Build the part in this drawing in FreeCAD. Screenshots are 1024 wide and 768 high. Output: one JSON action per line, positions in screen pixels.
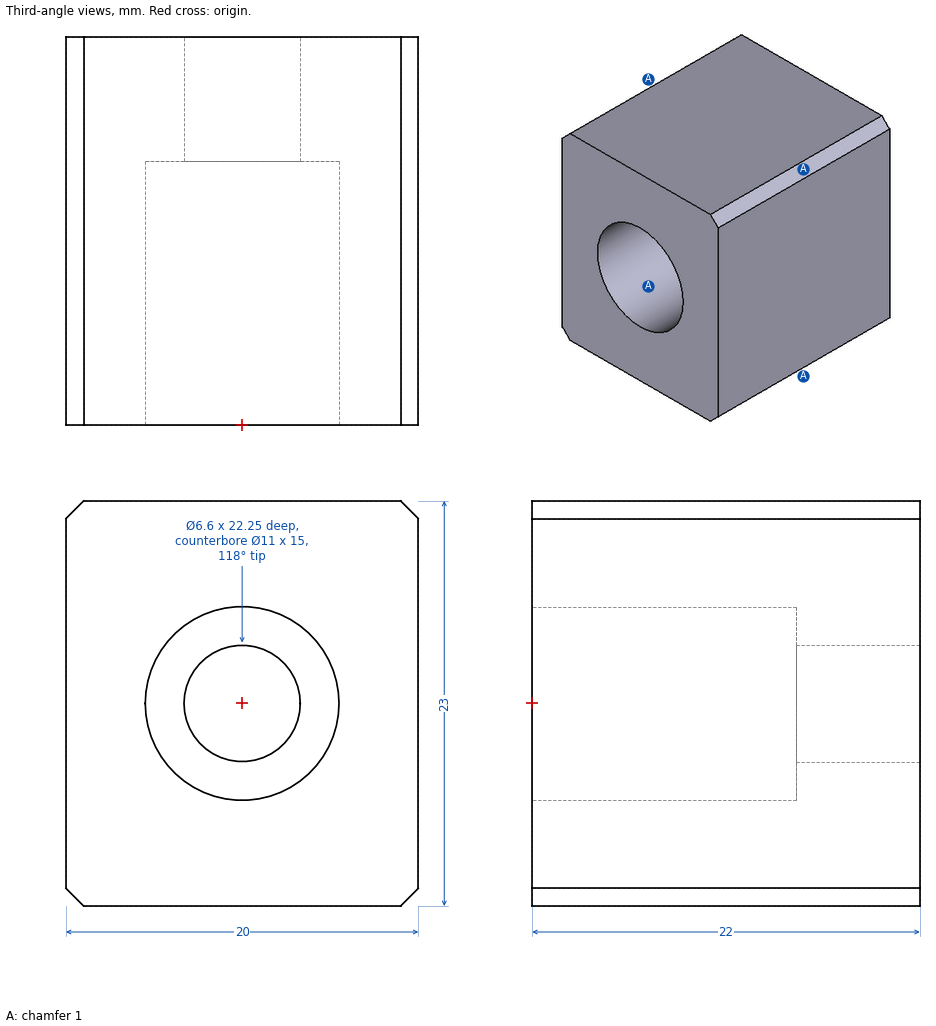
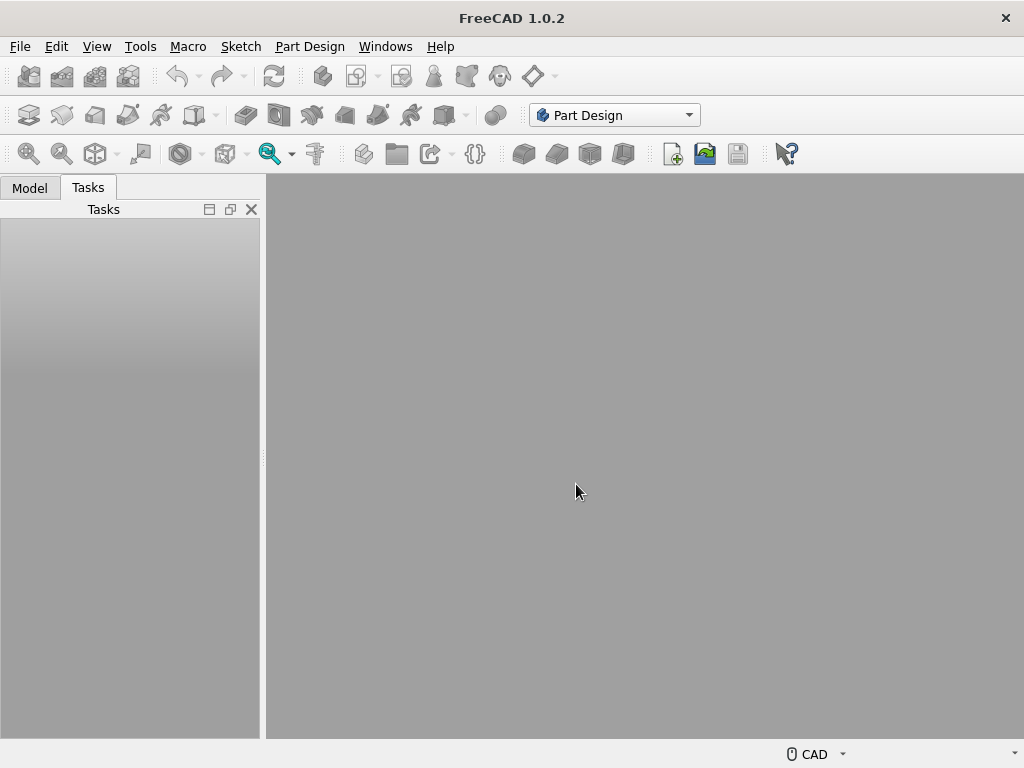
{"action": "key", "text": "ctrl+n"}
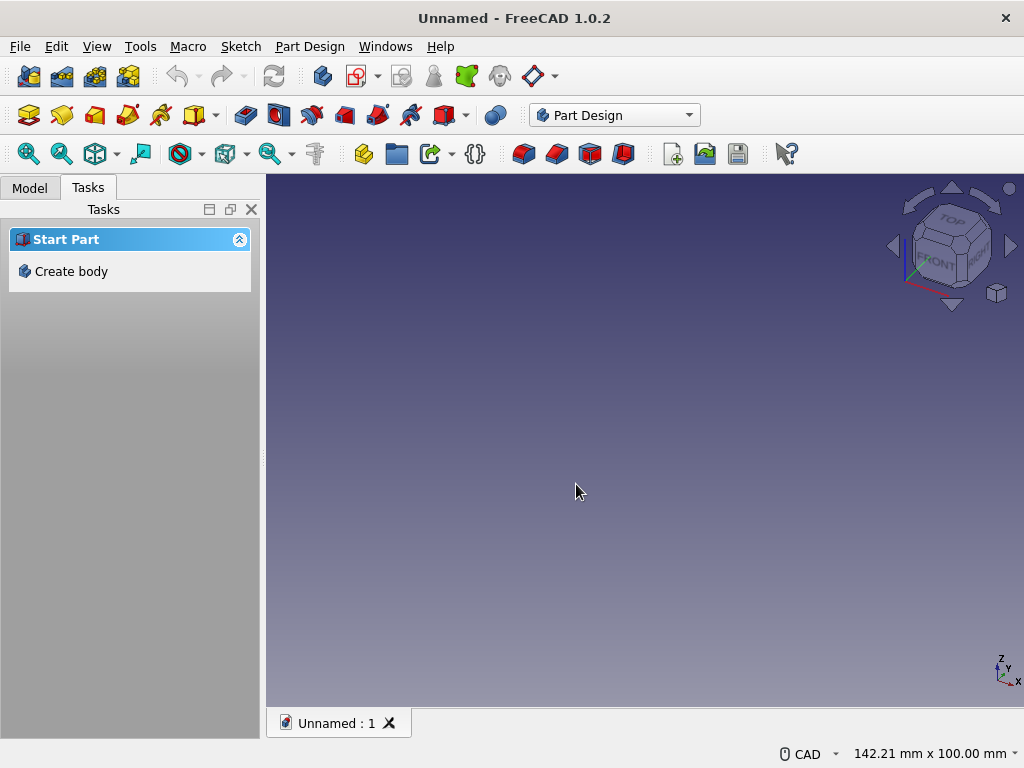
{"action": "left_click", "coordinate": [356, 76]}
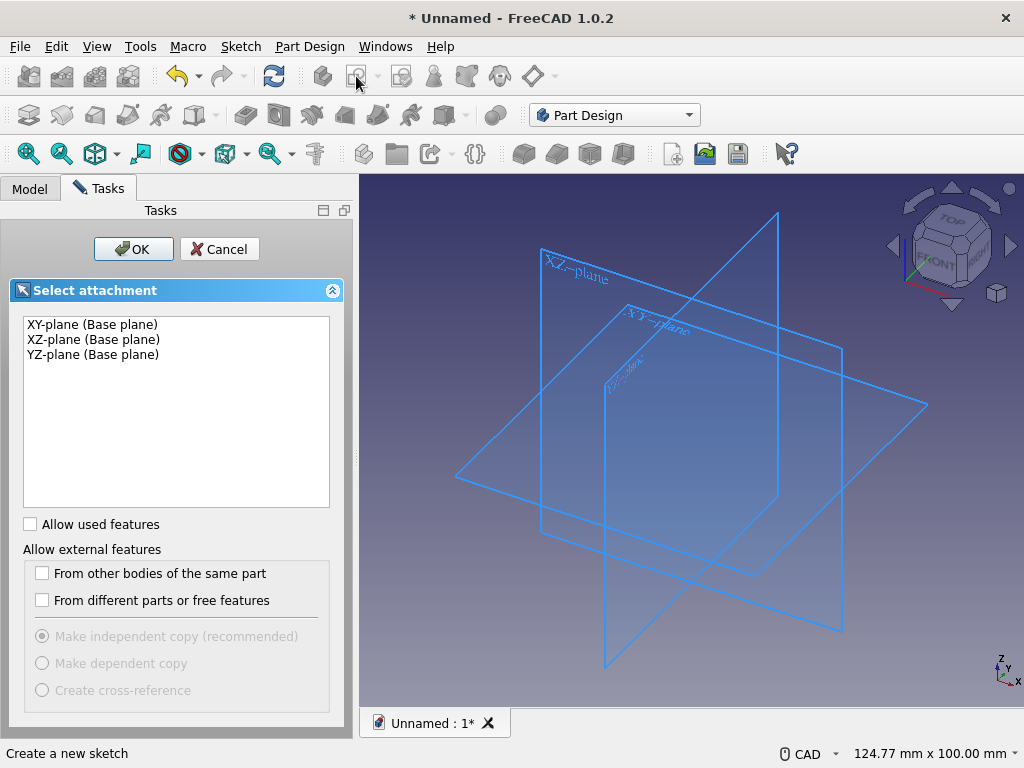
{"action": "left_click", "coordinate": [84, 340]}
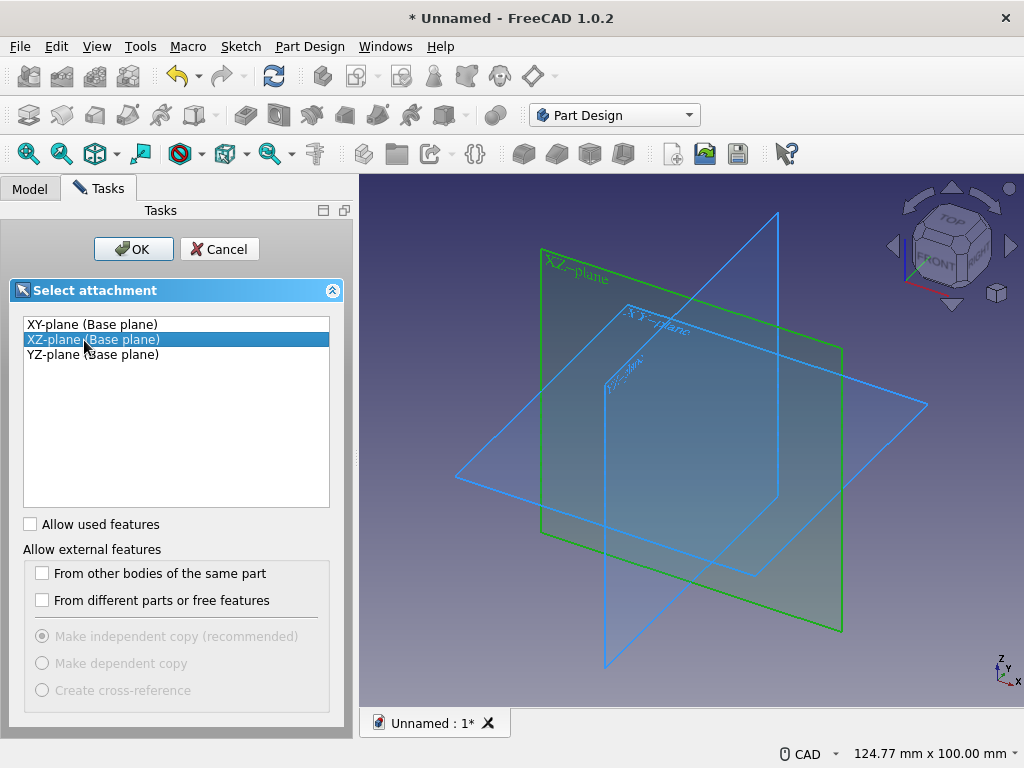
{"action": "left_click", "coordinate": [134, 249]}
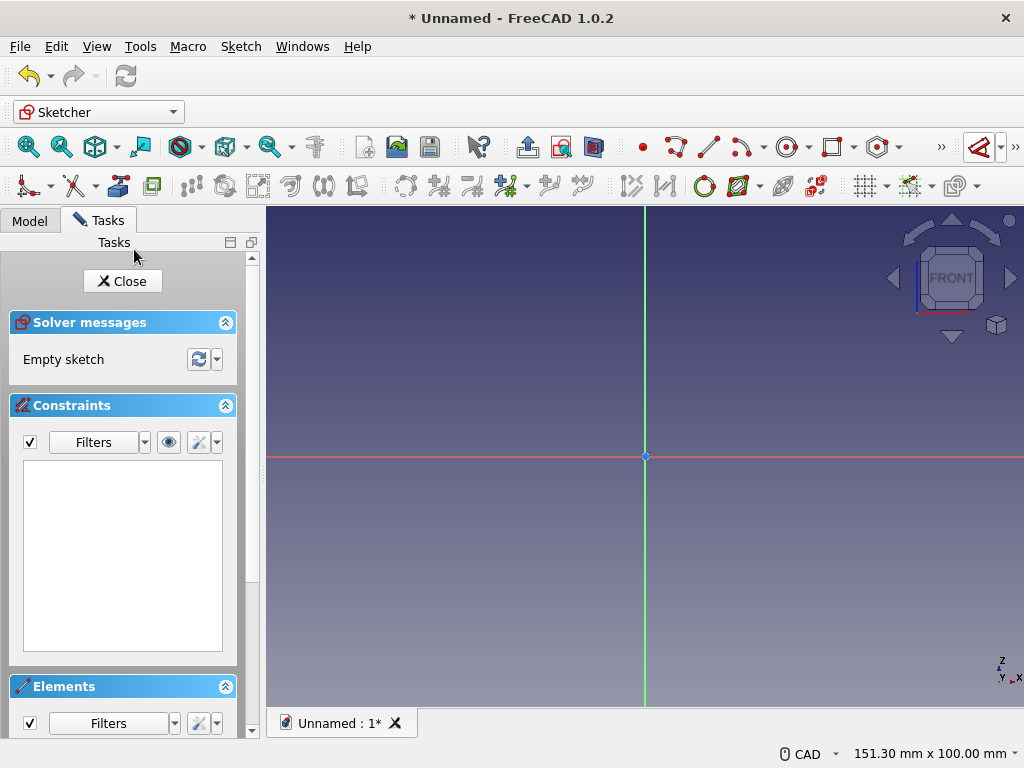
{"action": "scroll", "coordinate": [685, 456], "scroll_direction": "up", "scroll_amount": 5}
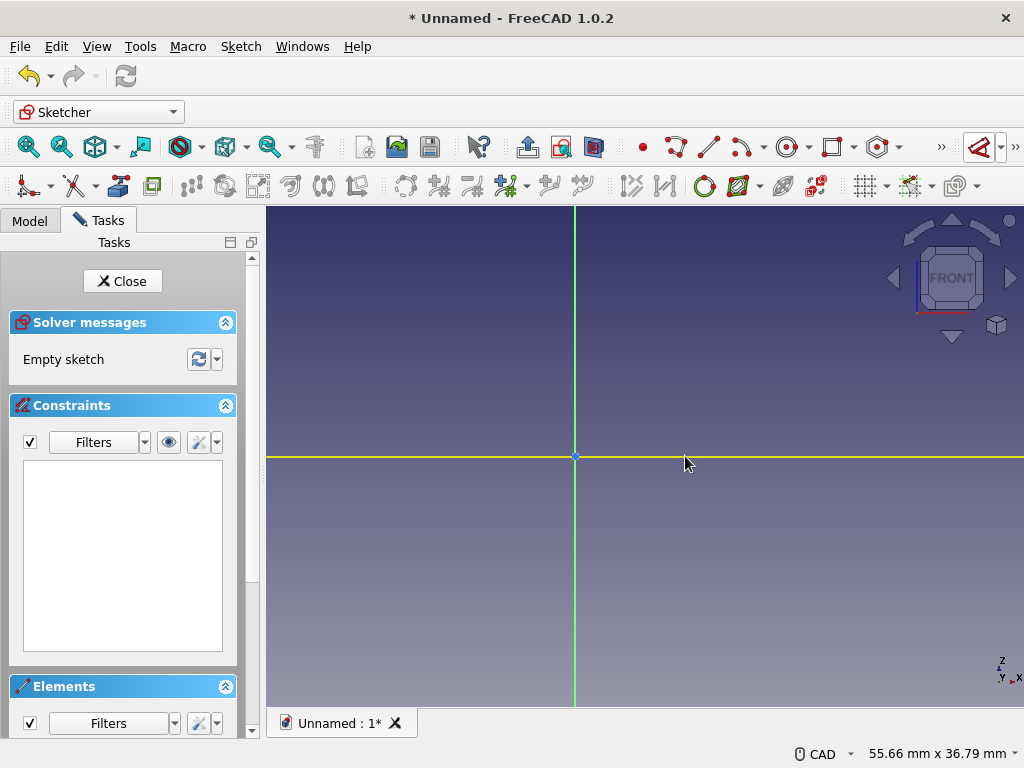
{"action": "key", "text": "g v"}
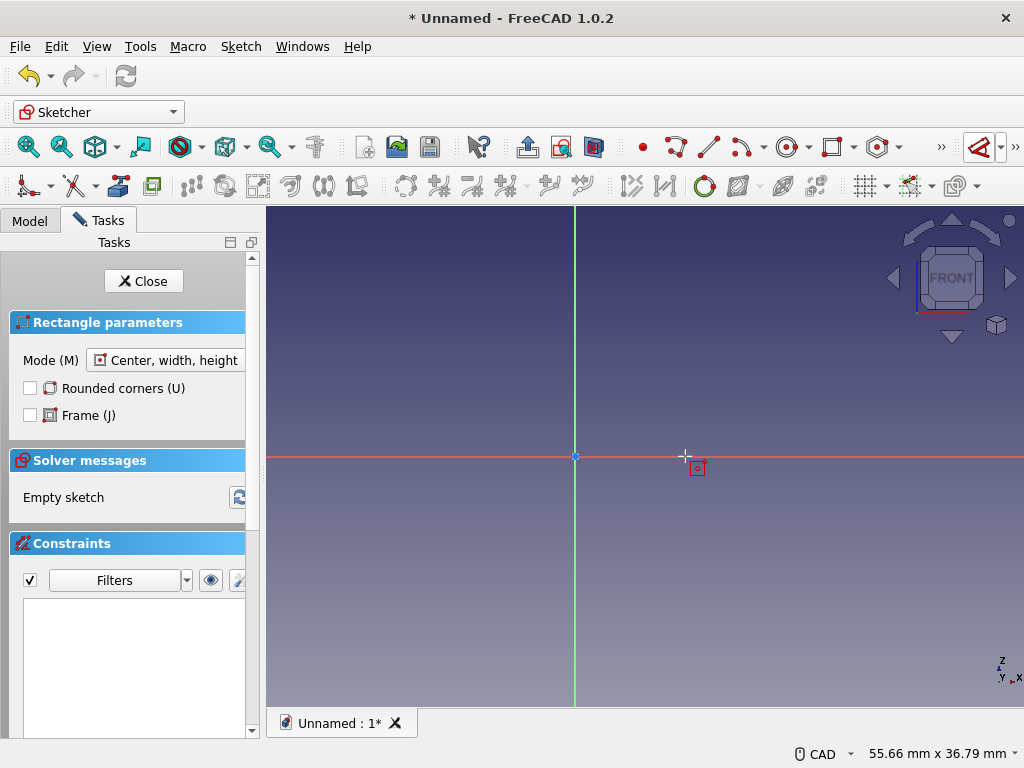
{"action": "left_click", "coordinate": [575, 456]}
{"action": "mouse_move", "coordinate": [712, 300]}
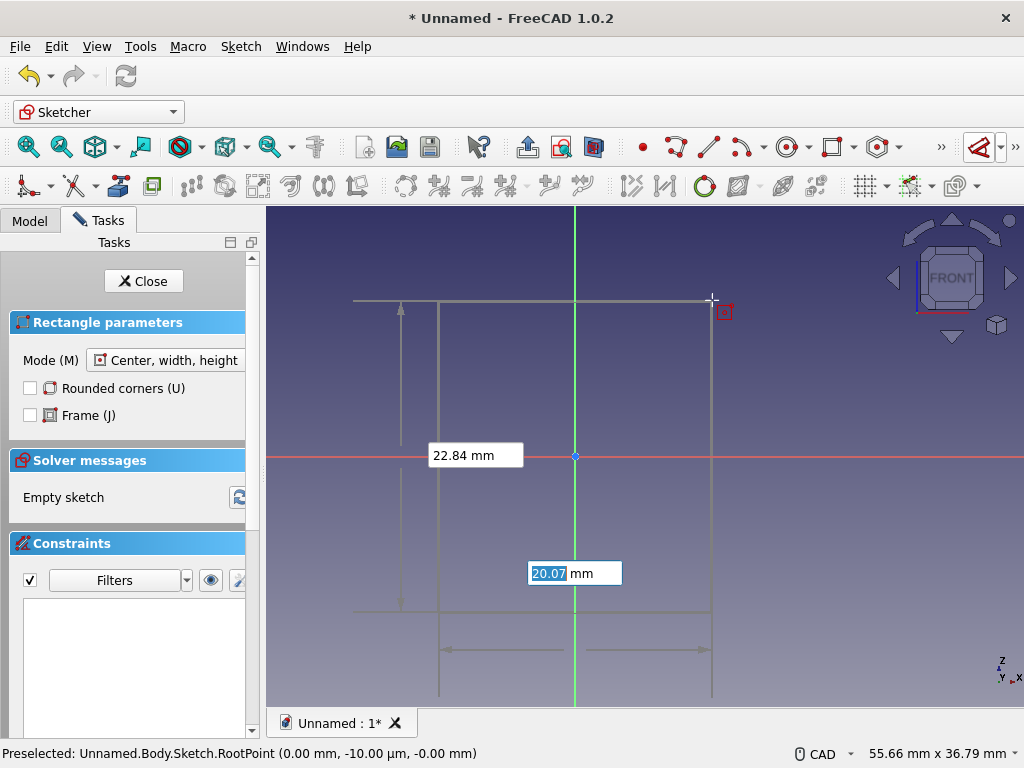
{"action": "type", "text": "20"}
{"action": "key", "text": "Tab"}
{"action": "type", "text": "23"}
{"action": "key", "text": "Return"}
{"action": "key", "text": "Escape"}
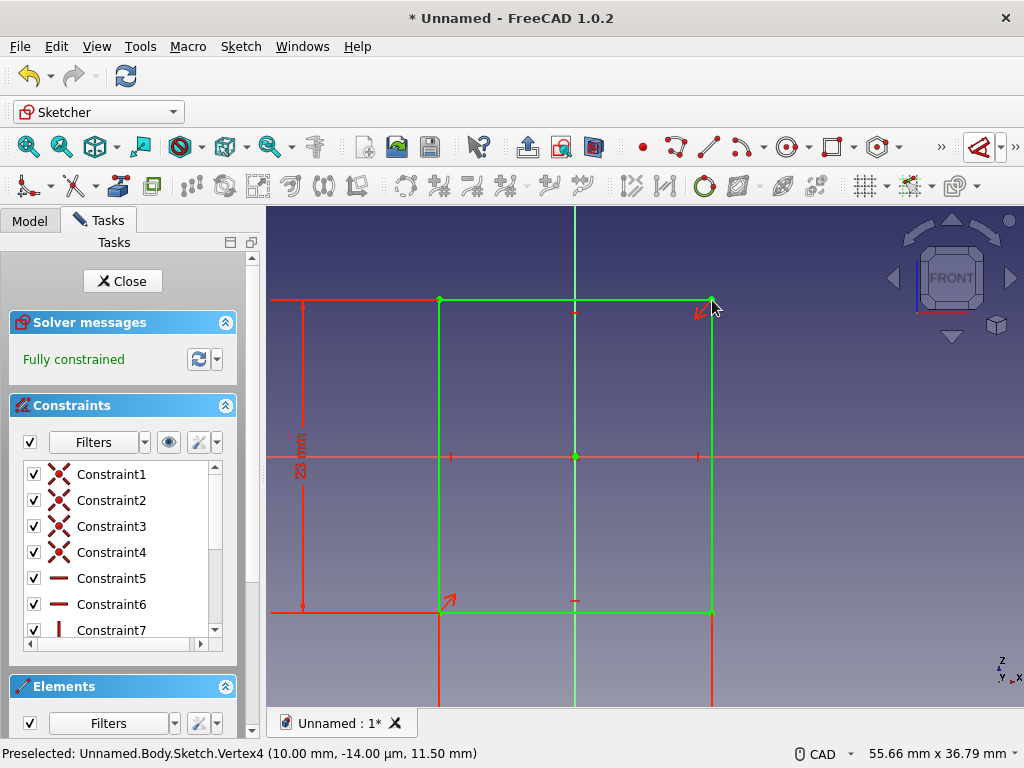
{"action": "left_click", "coordinate": [123, 281]}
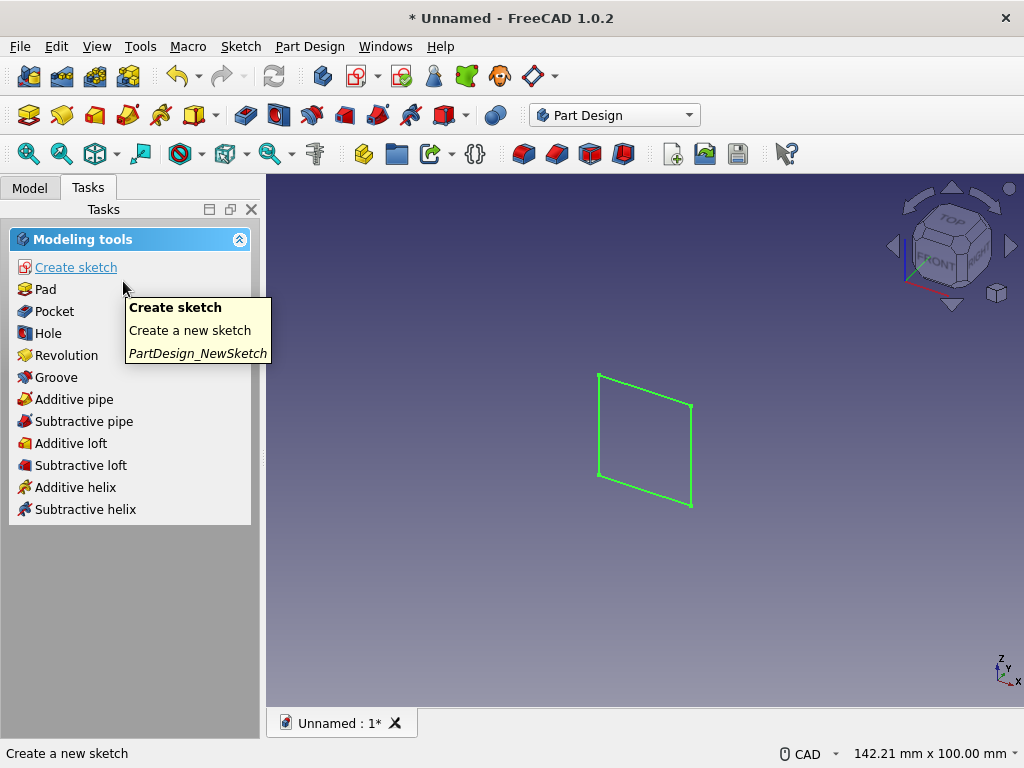
{"action": "left_click", "coordinate": [29, 116]}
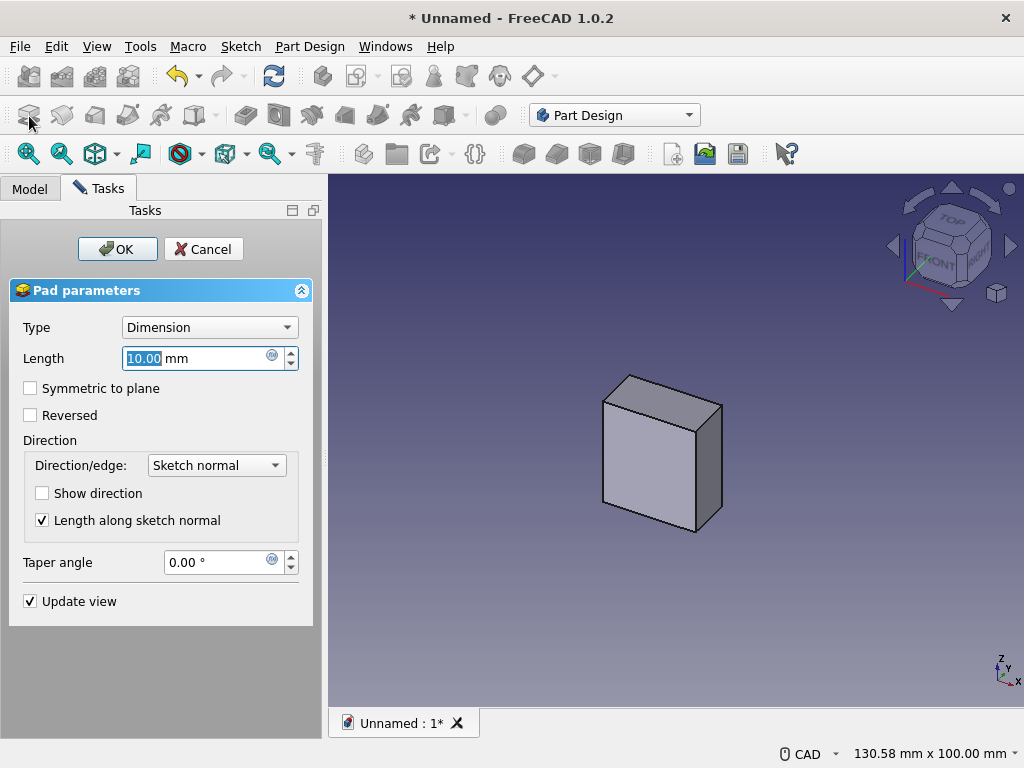
{"action": "type", "text": "22"}
{"action": "key", "text": "Tab"}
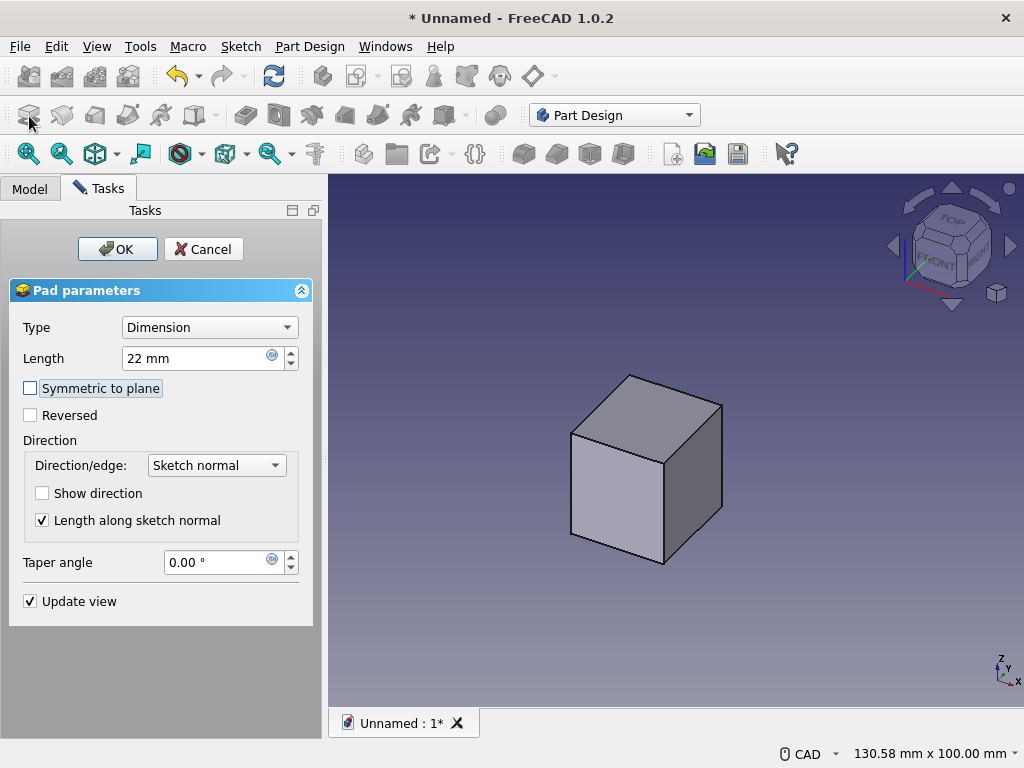
{"action": "left_click", "coordinate": [31, 415]}